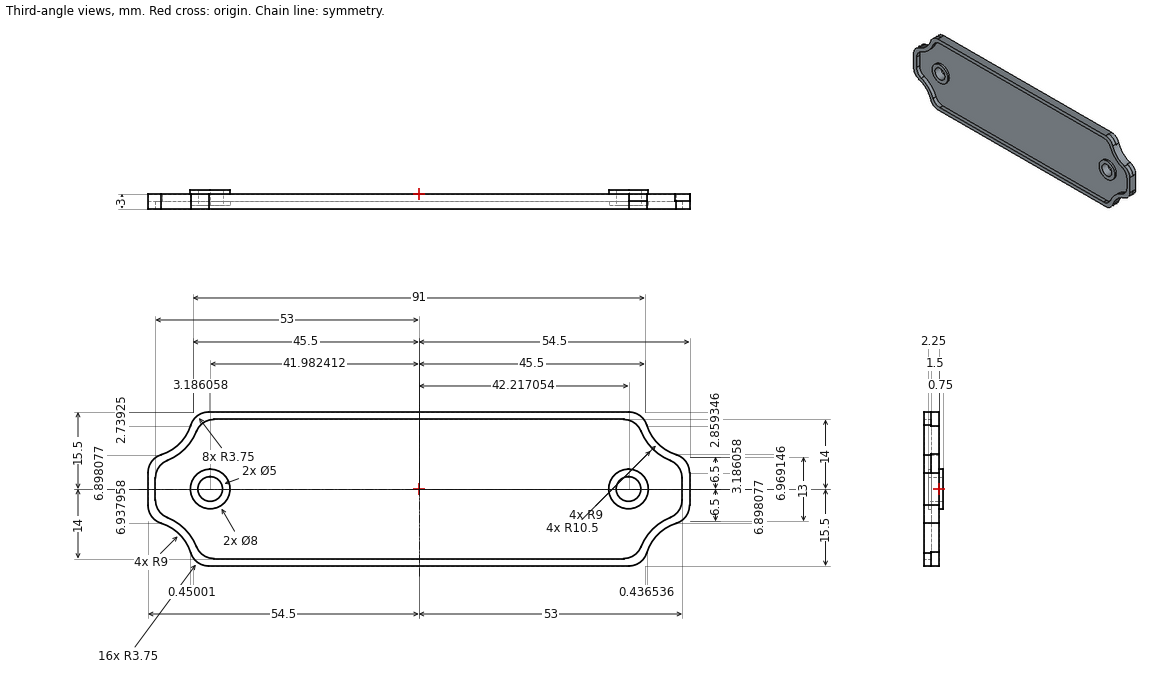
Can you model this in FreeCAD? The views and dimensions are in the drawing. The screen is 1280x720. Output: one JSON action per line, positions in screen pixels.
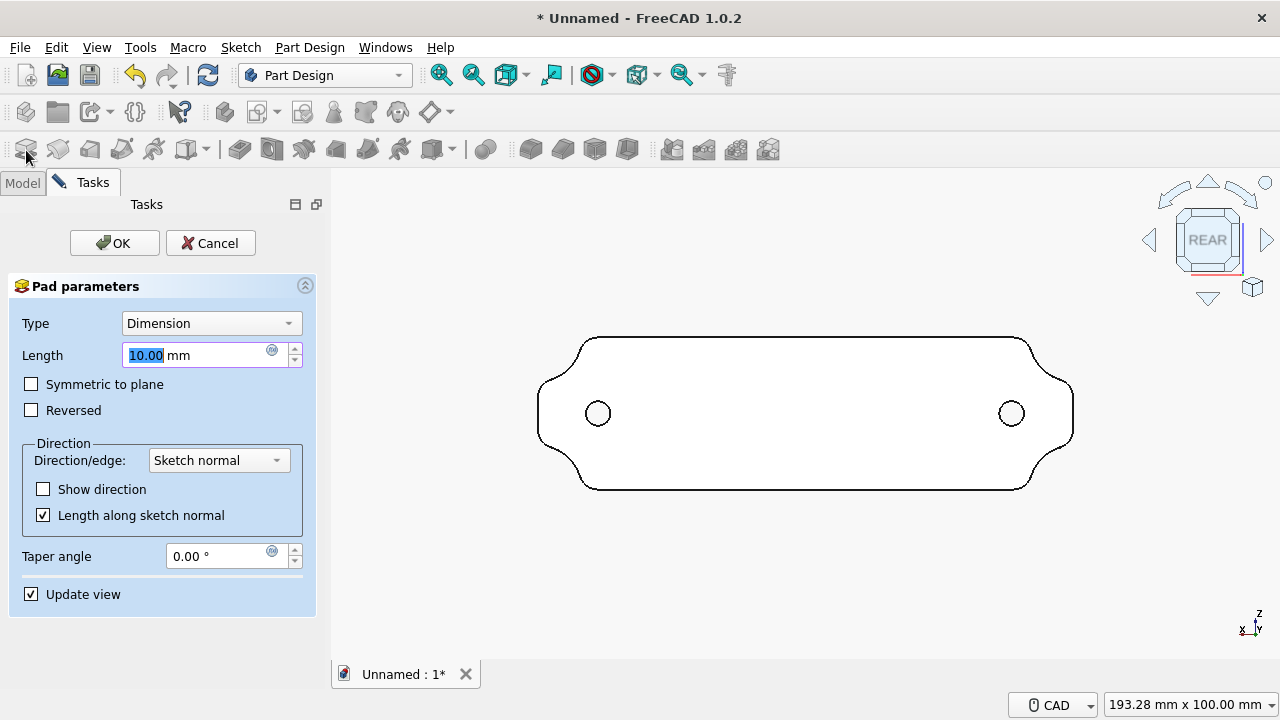
{"action": "left_click", "coordinate": [212, 324]}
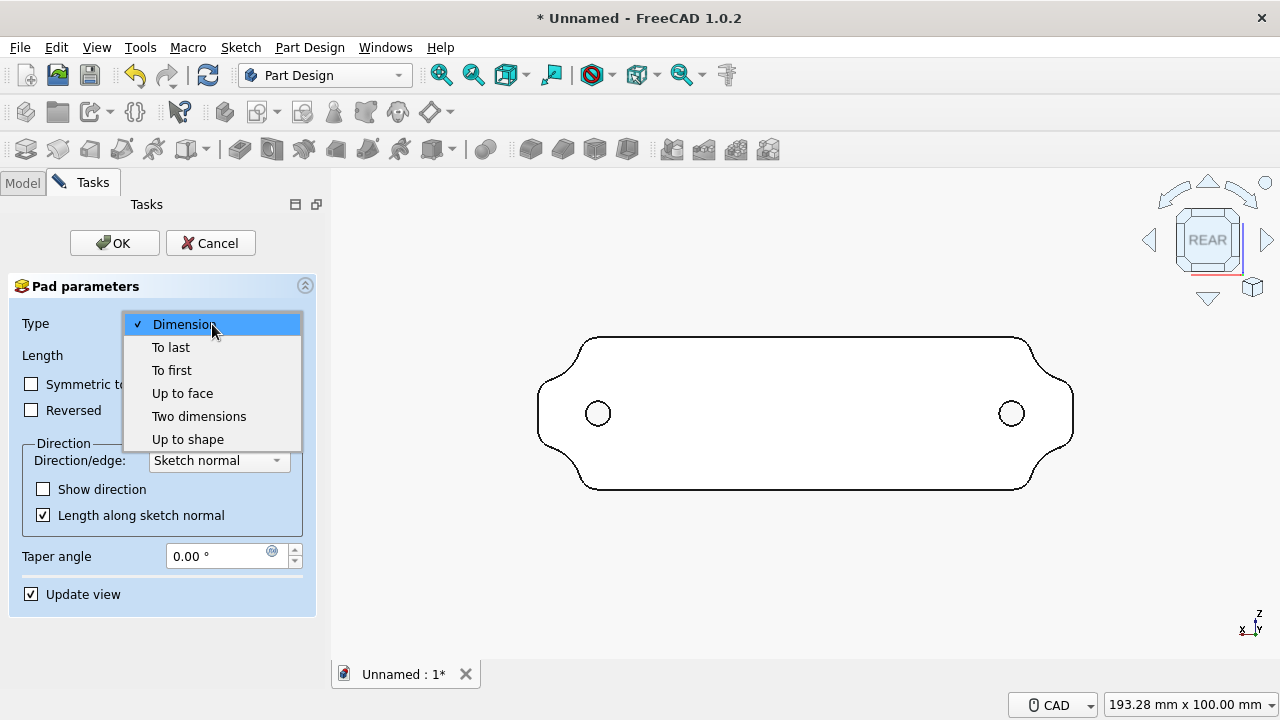
{"action": "left_click", "coordinate": [212, 416]}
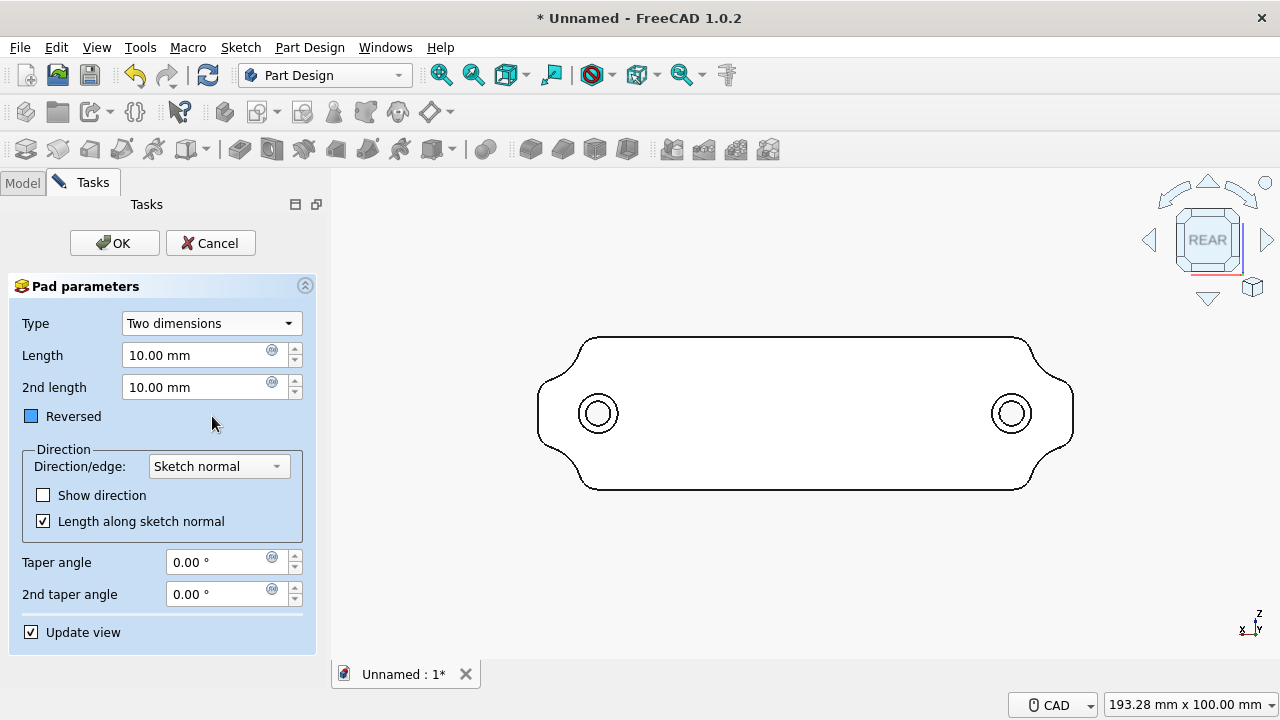
{"action": "triple_click", "coordinate": [204, 355]}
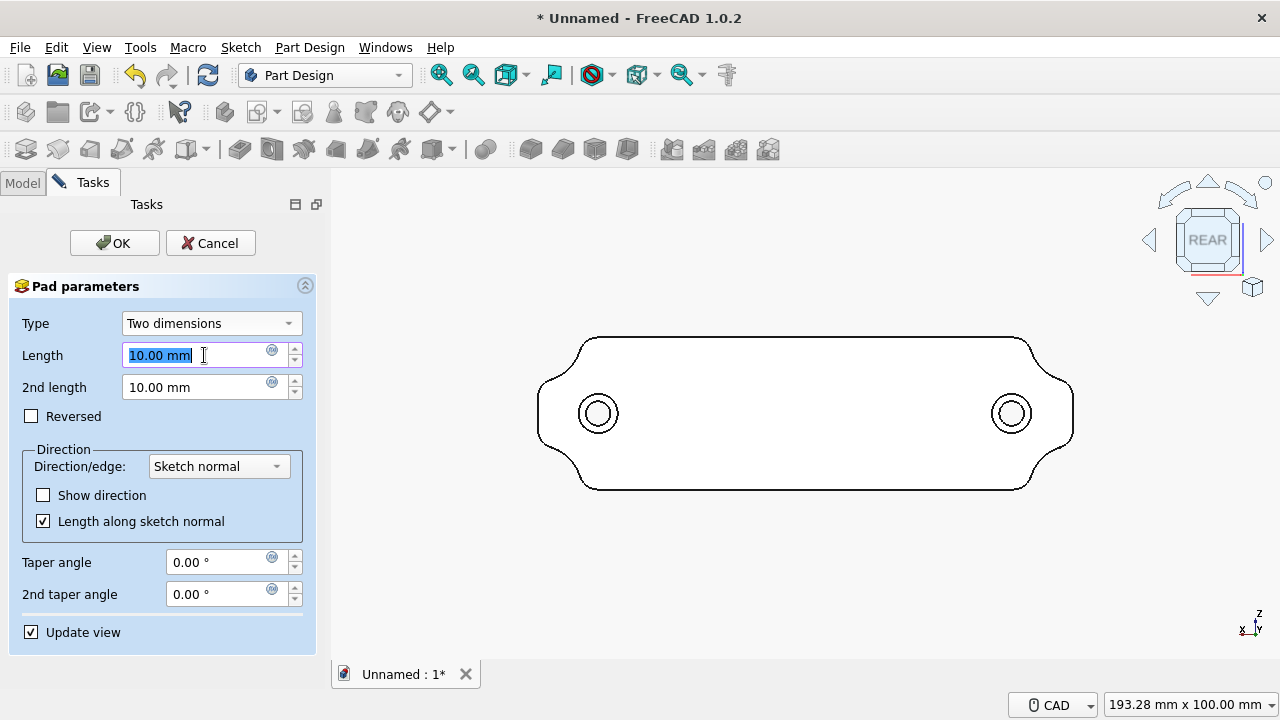
{"action": "type", "text": "0.75"}
{"action": "key", "text": "Tab"}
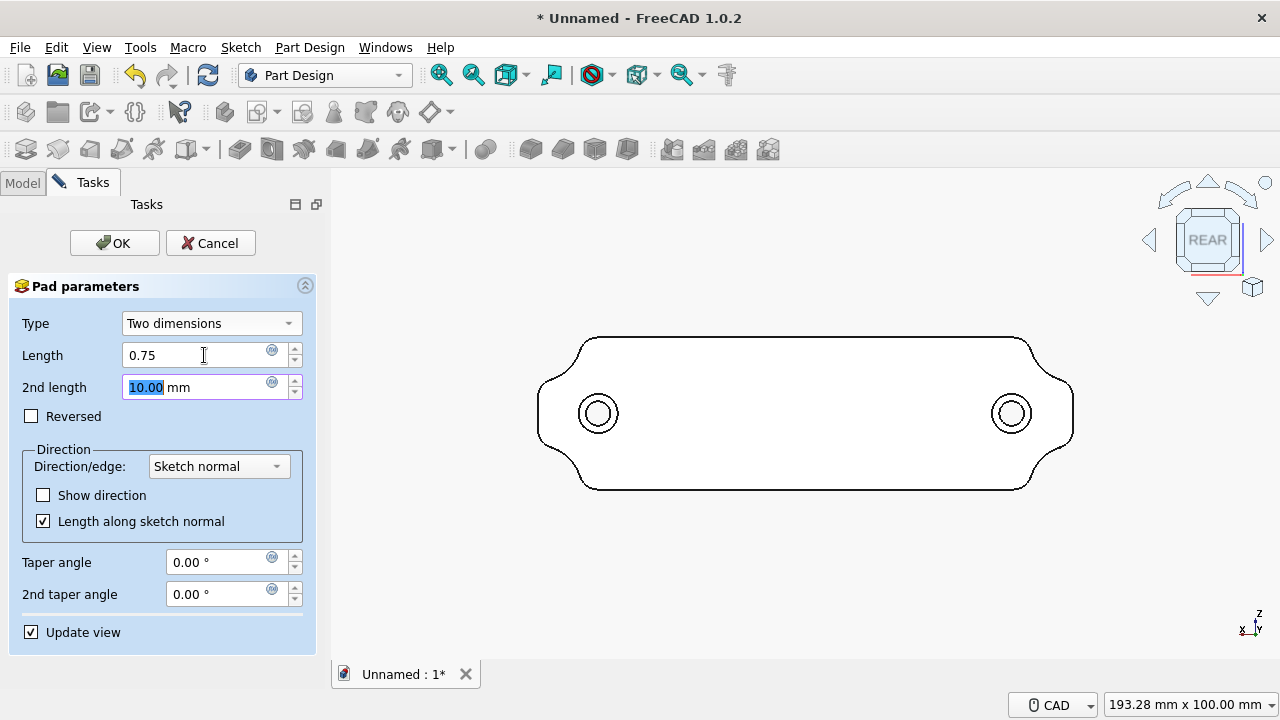
{"action": "type", "text": "2.25"}
{"action": "key", "text": "Tab"}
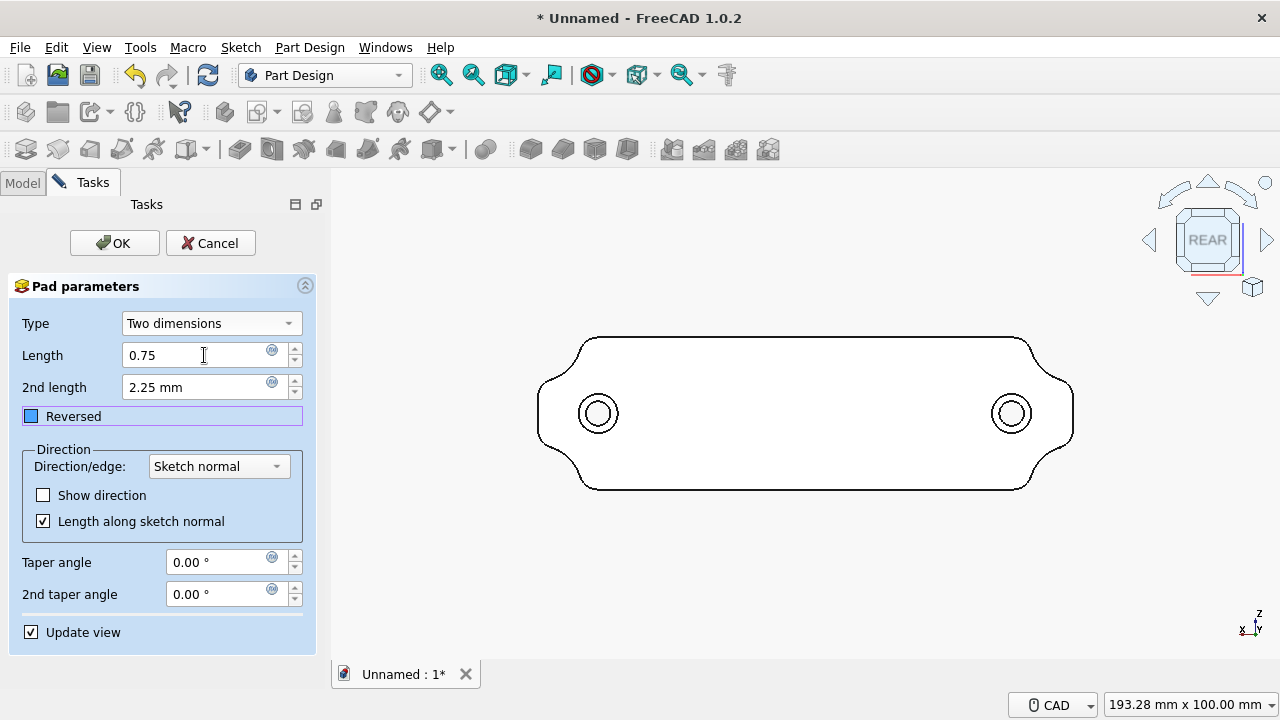
{"action": "left_click", "coordinate": [30, 416]}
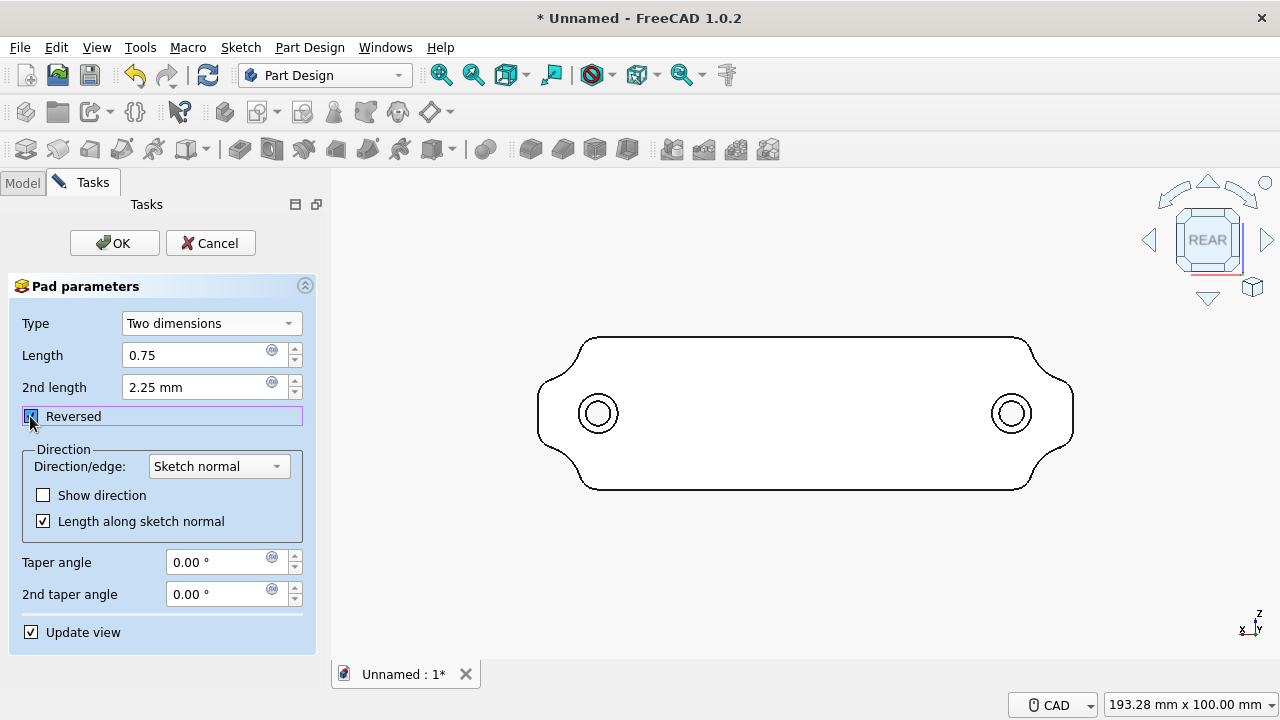
{"action": "left_click", "coordinate": [115, 243]}